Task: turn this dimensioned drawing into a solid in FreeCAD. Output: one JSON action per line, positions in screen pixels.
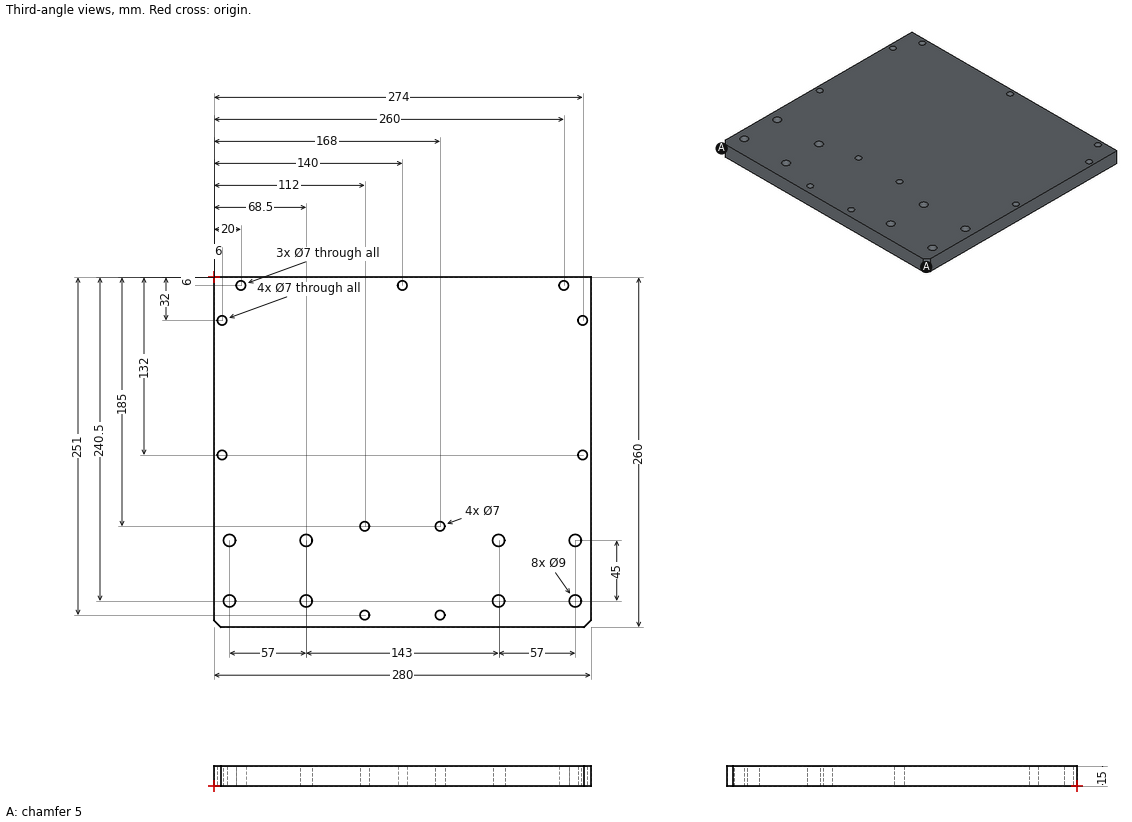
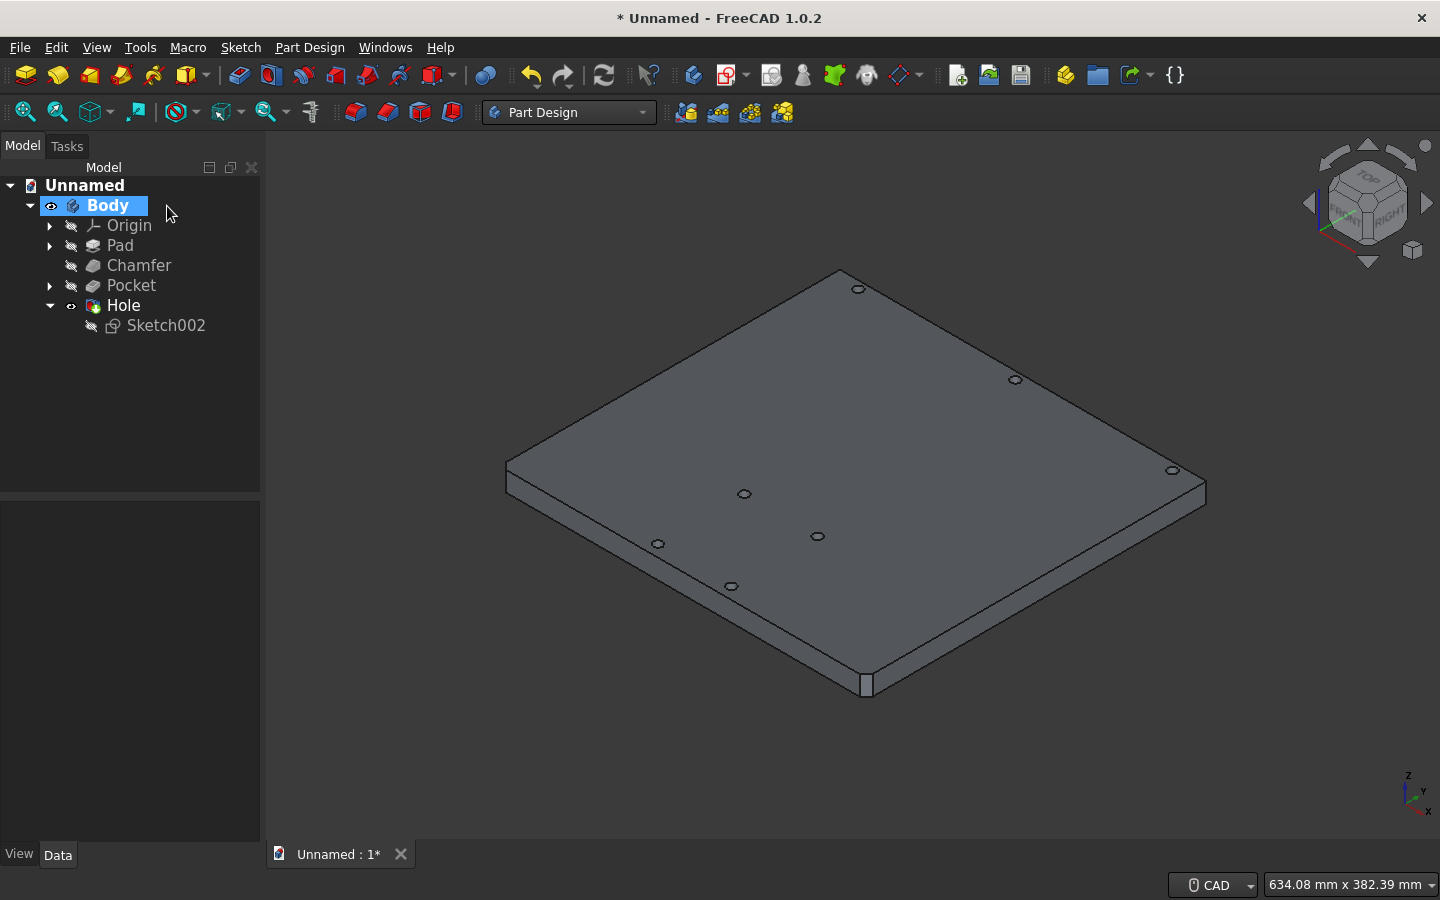
{"action": "left_click", "coordinate": [726, 76]}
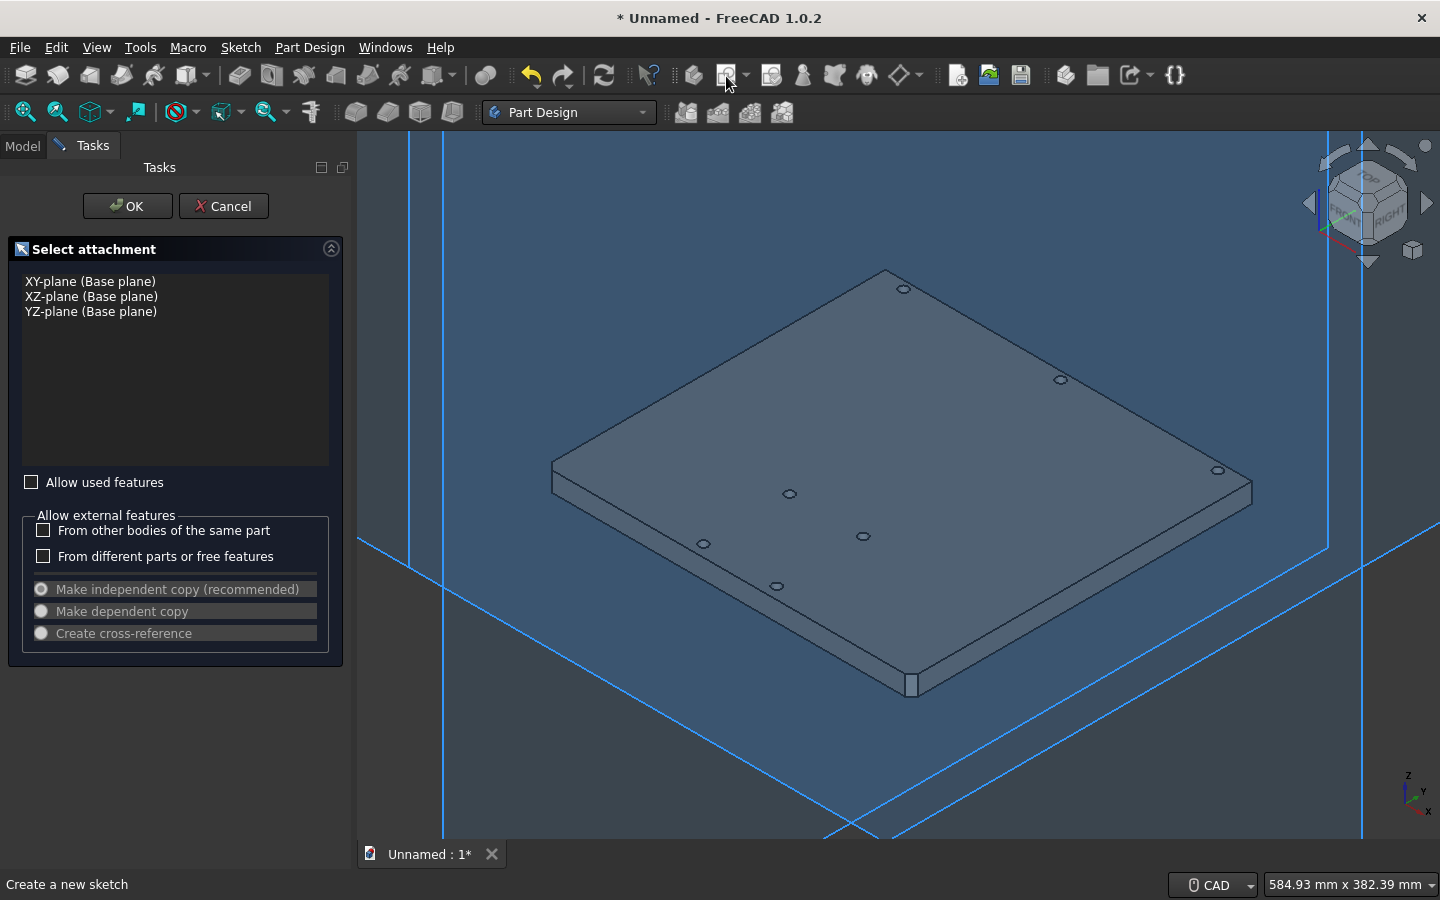
{"action": "left_click", "coordinate": [82, 282]}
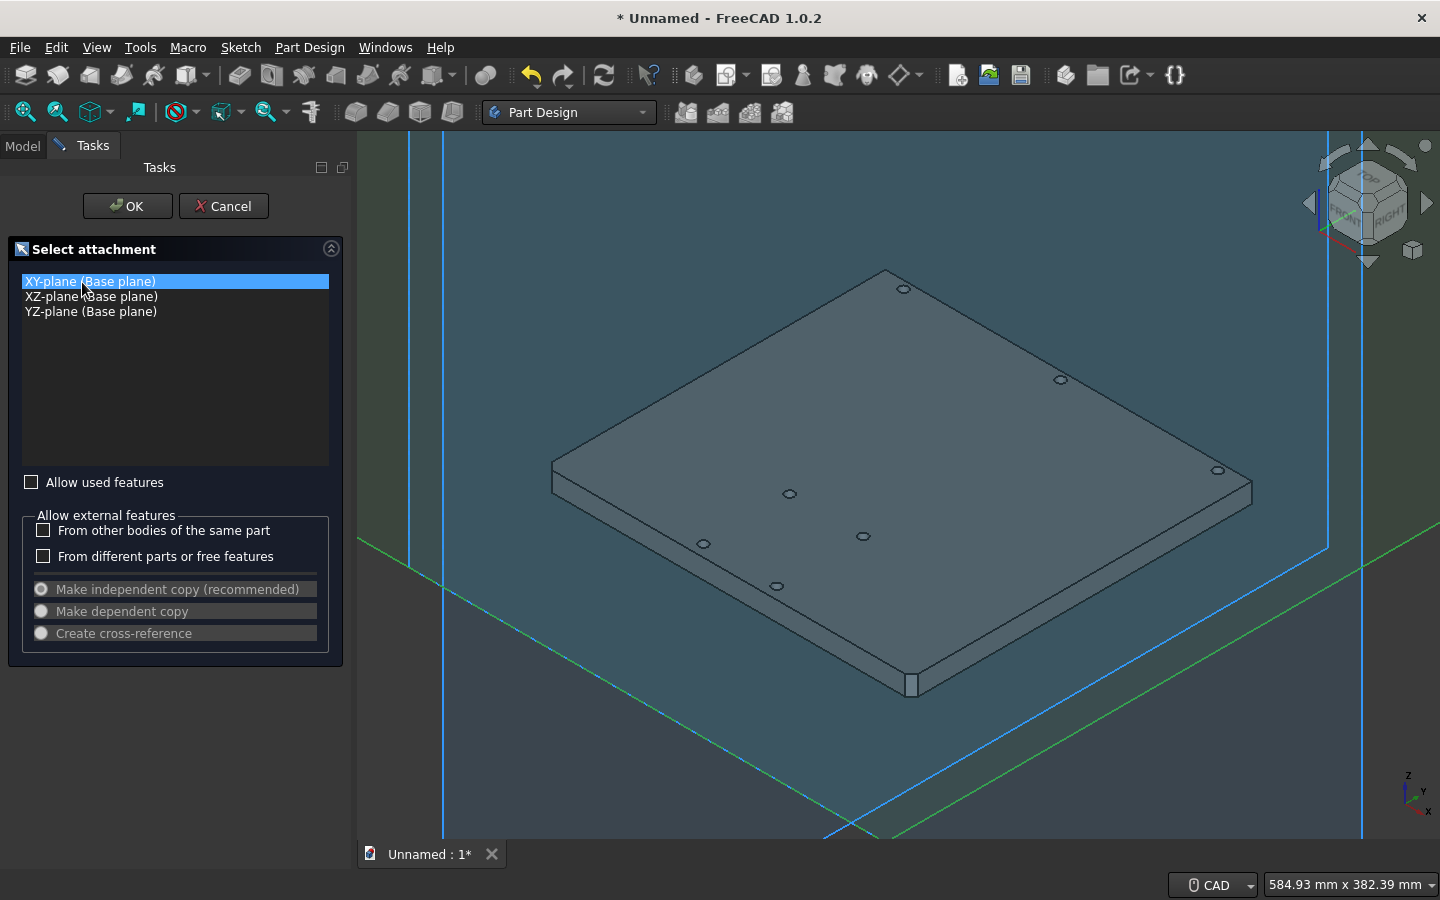
{"action": "left_click", "coordinate": [128, 206]}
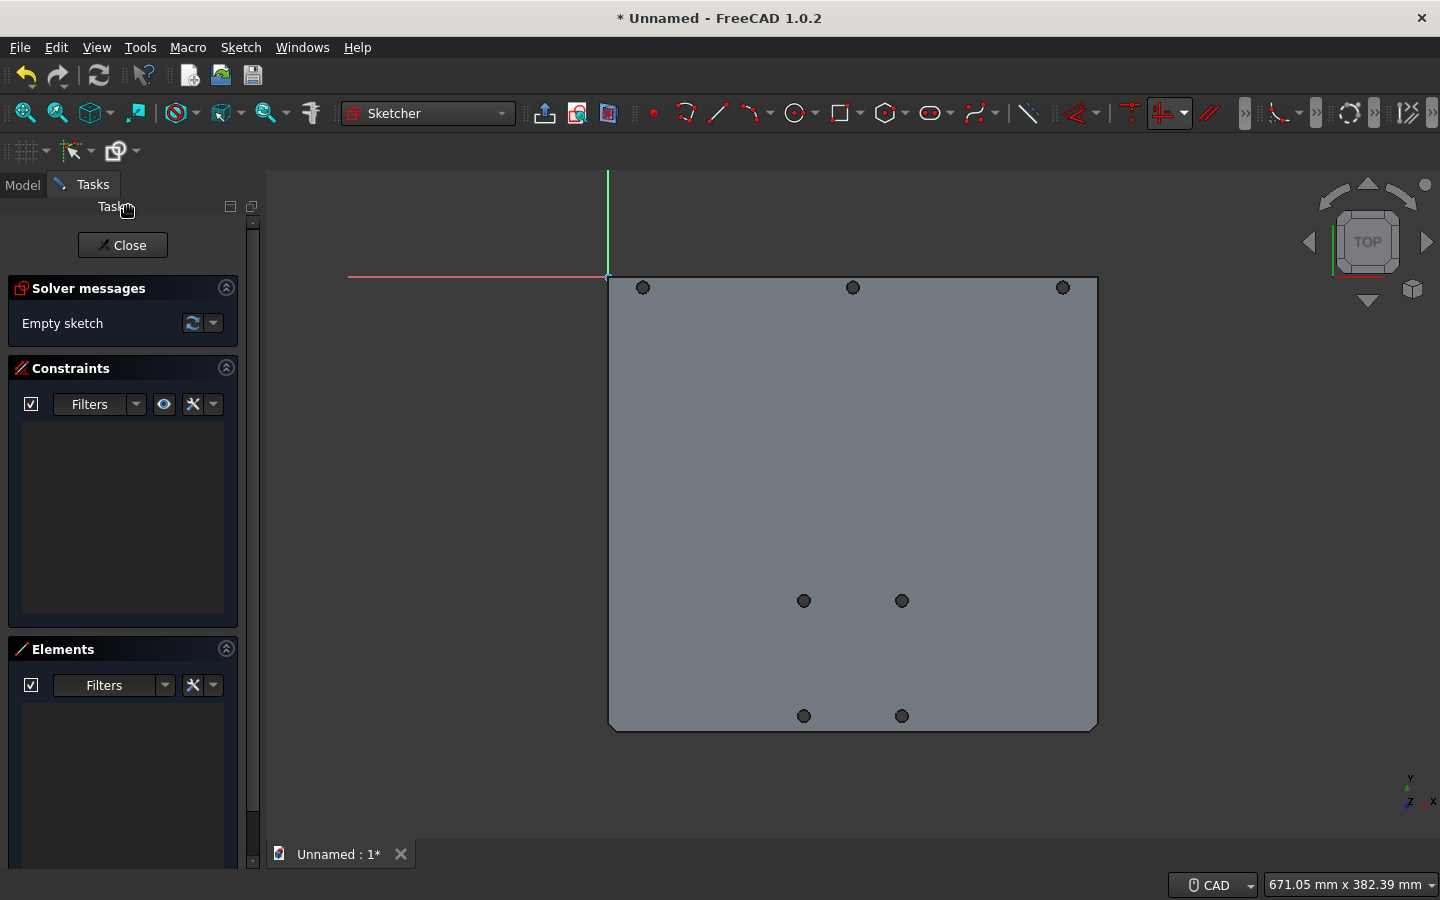
{"action": "left_click", "coordinate": [610, 114]}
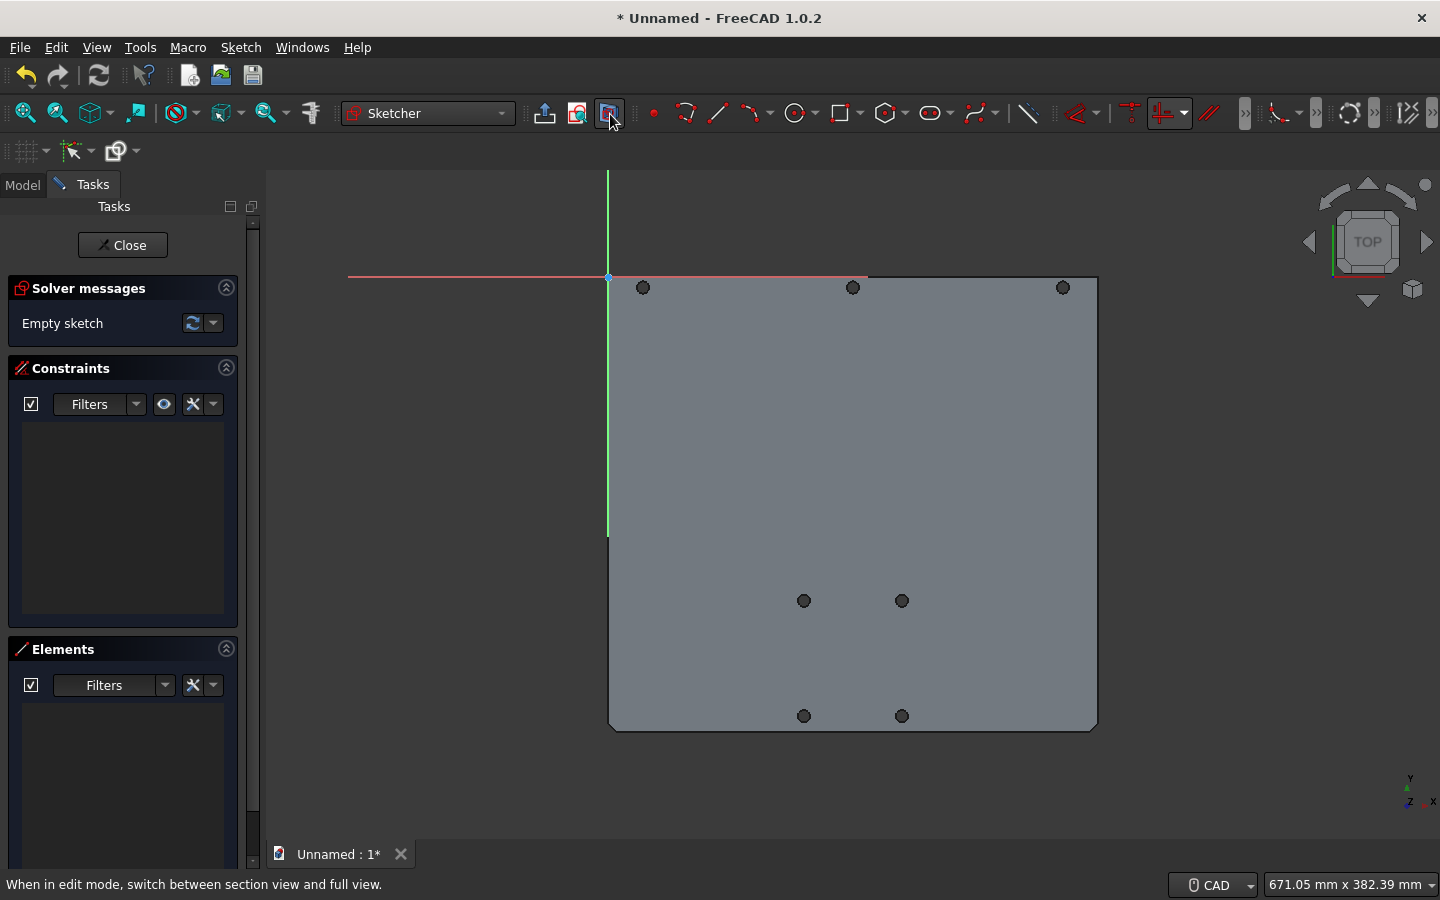
{"action": "left_click", "coordinate": [796, 114]}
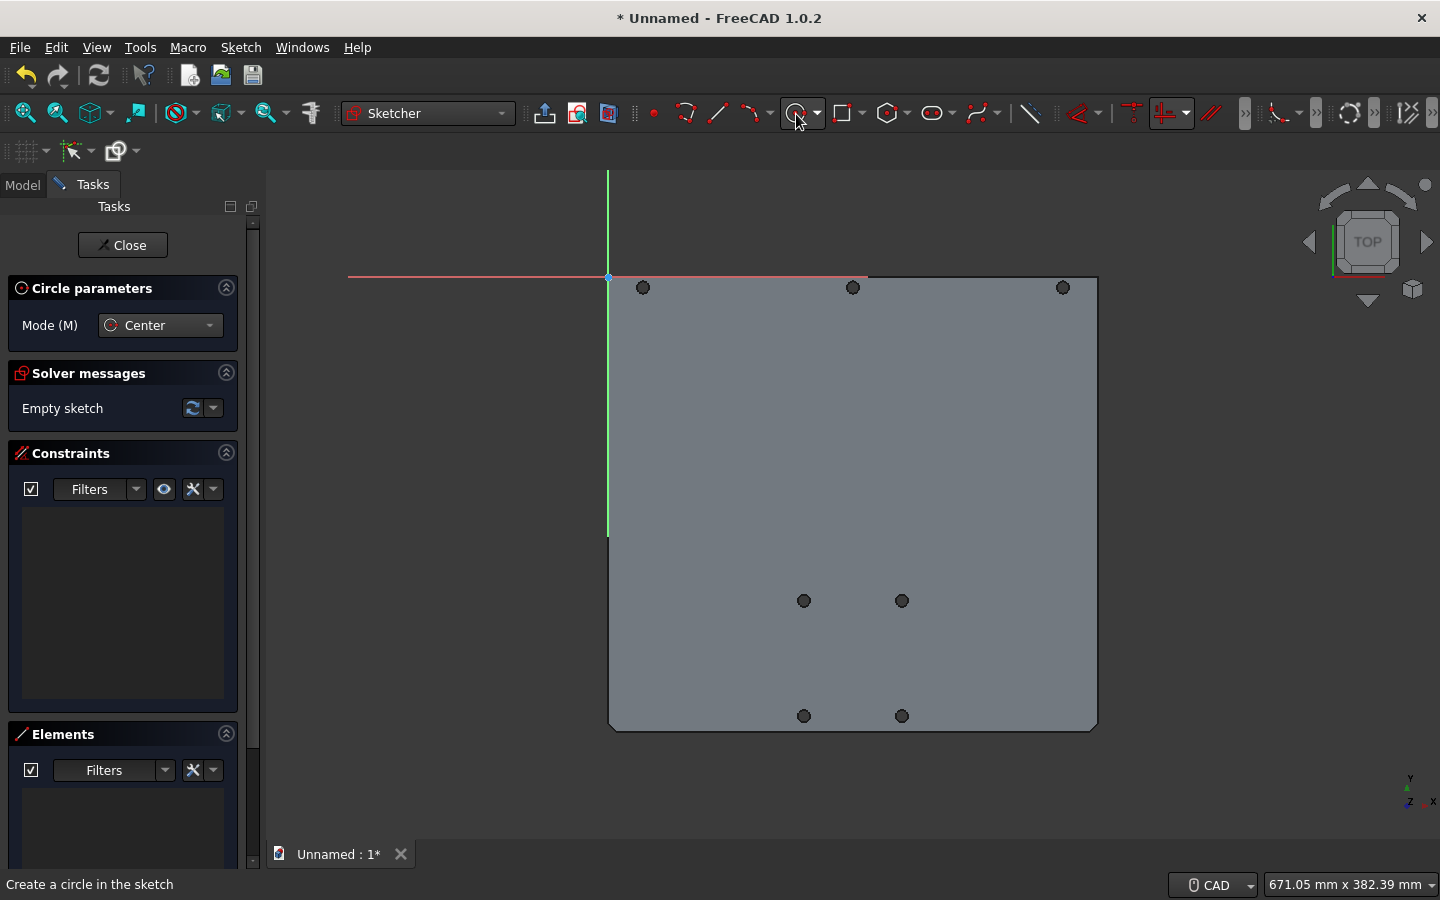
{"action": "scroll", "coordinate": [1078, 698], "scroll_direction": "up", "scroll_amount": 6}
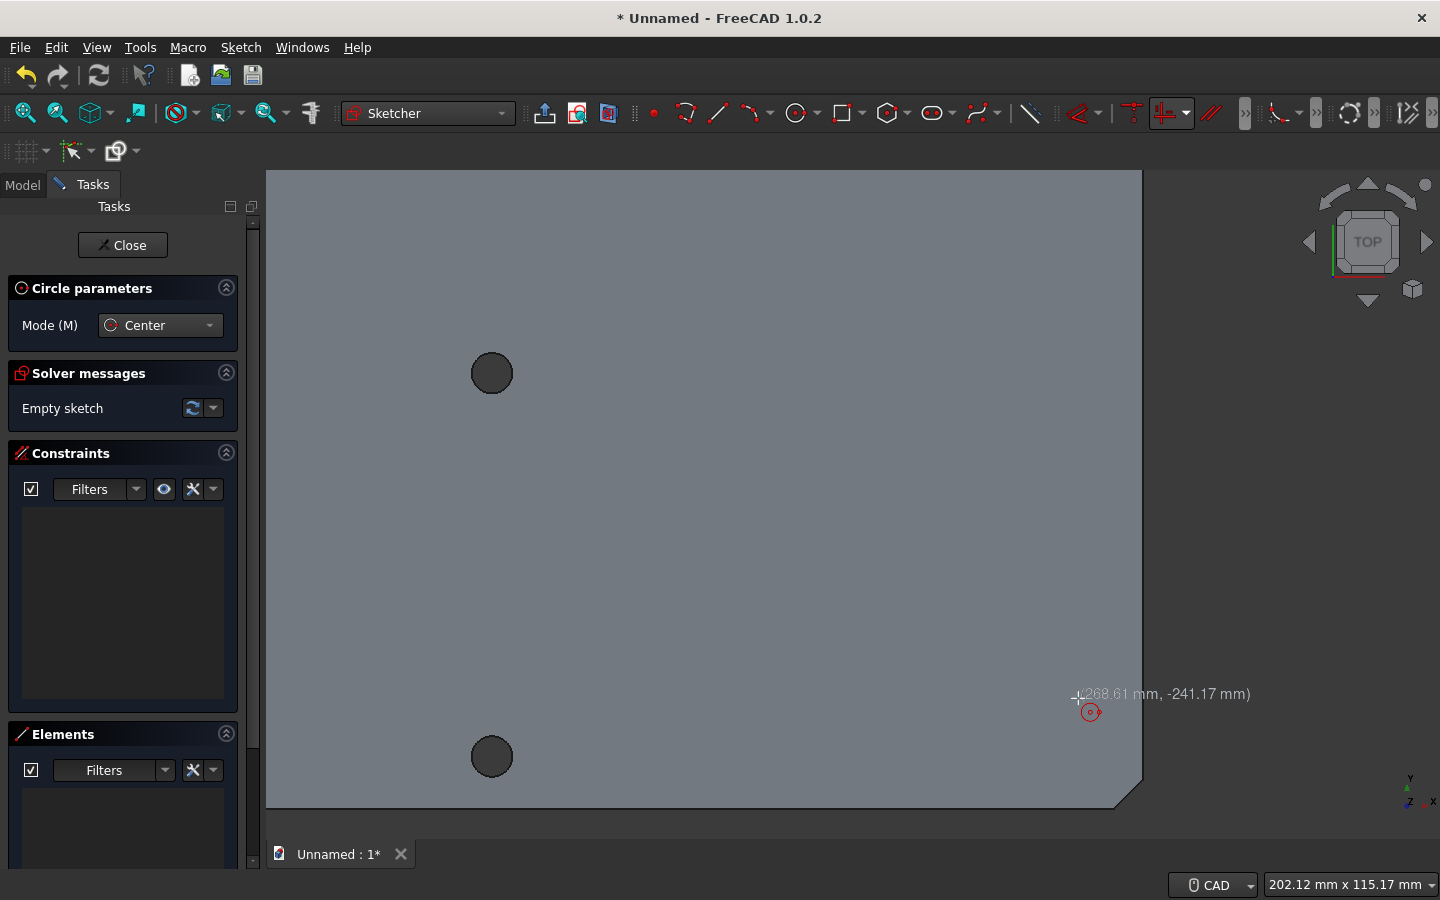
{"action": "left_click", "coordinate": [1076, 696]}
{"action": "mouse_move", "coordinate": [1094, 677]}